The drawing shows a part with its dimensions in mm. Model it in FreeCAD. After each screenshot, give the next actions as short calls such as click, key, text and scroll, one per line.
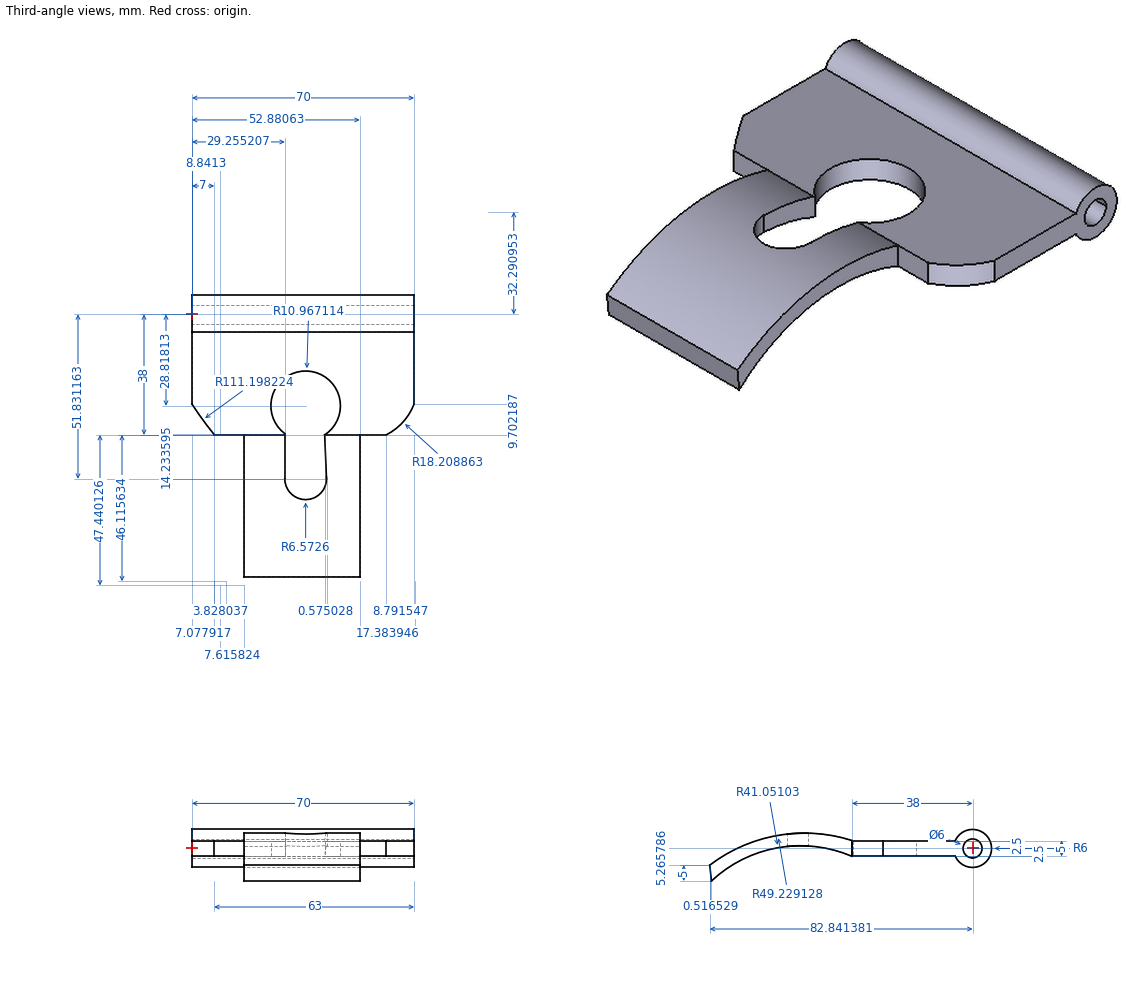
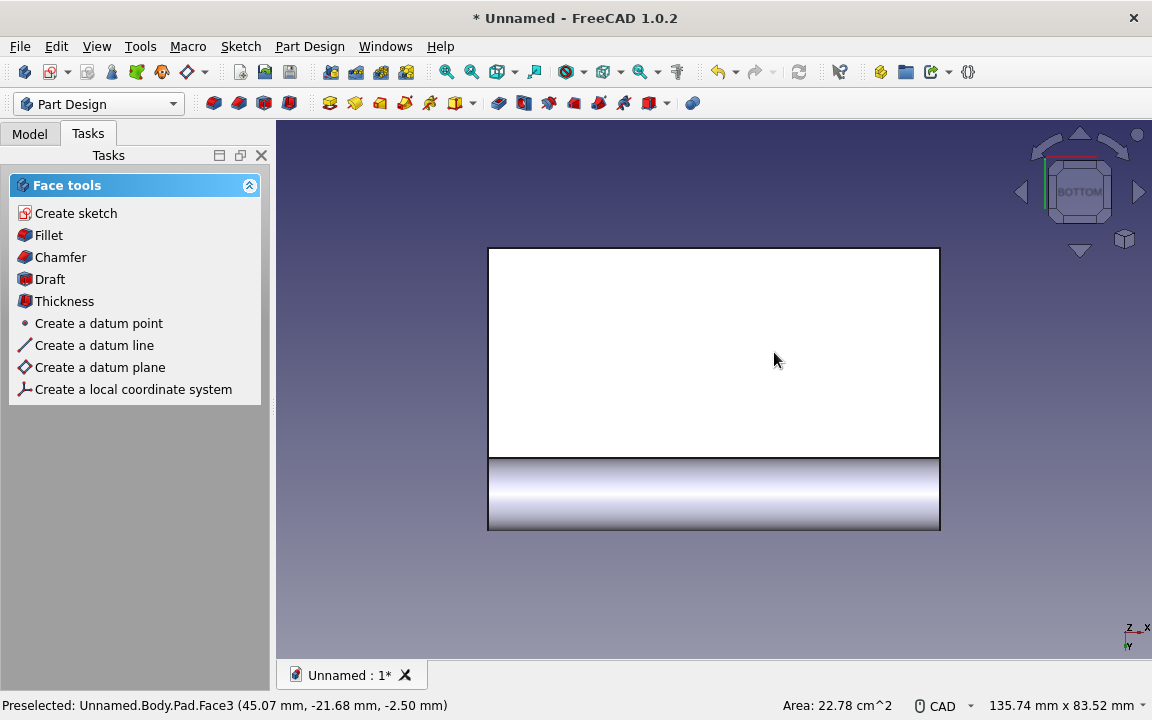
click(50, 72)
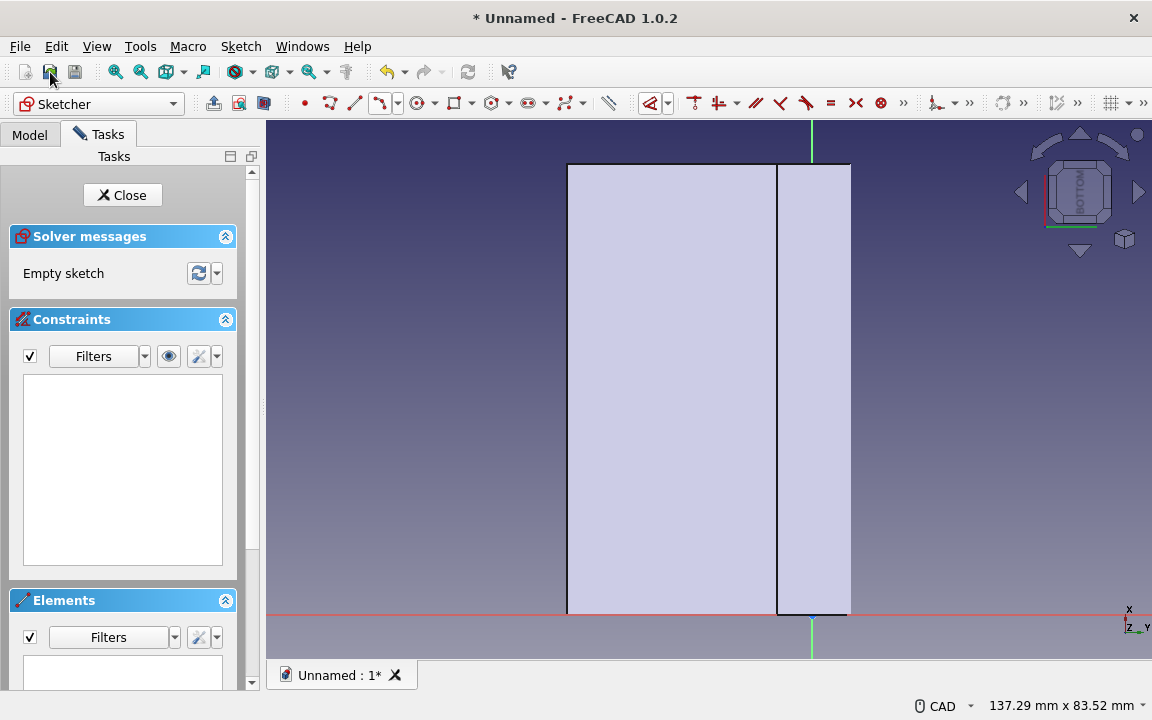
click(264, 104)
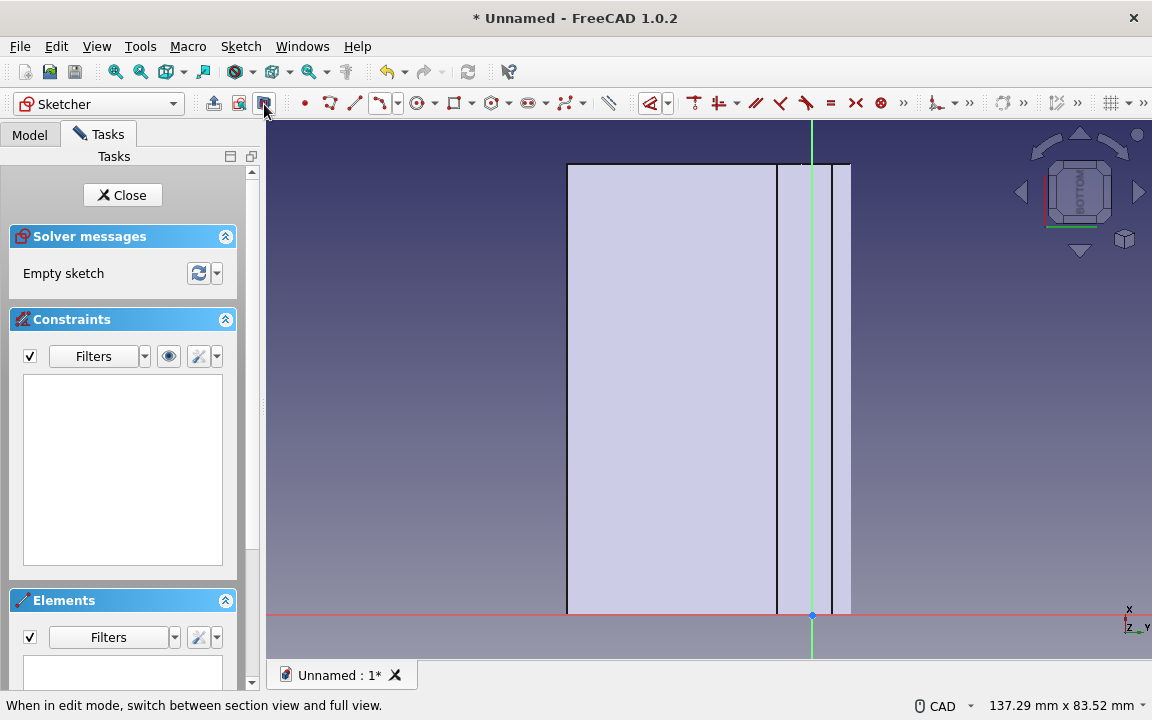
scroll(418, 389, down, 1)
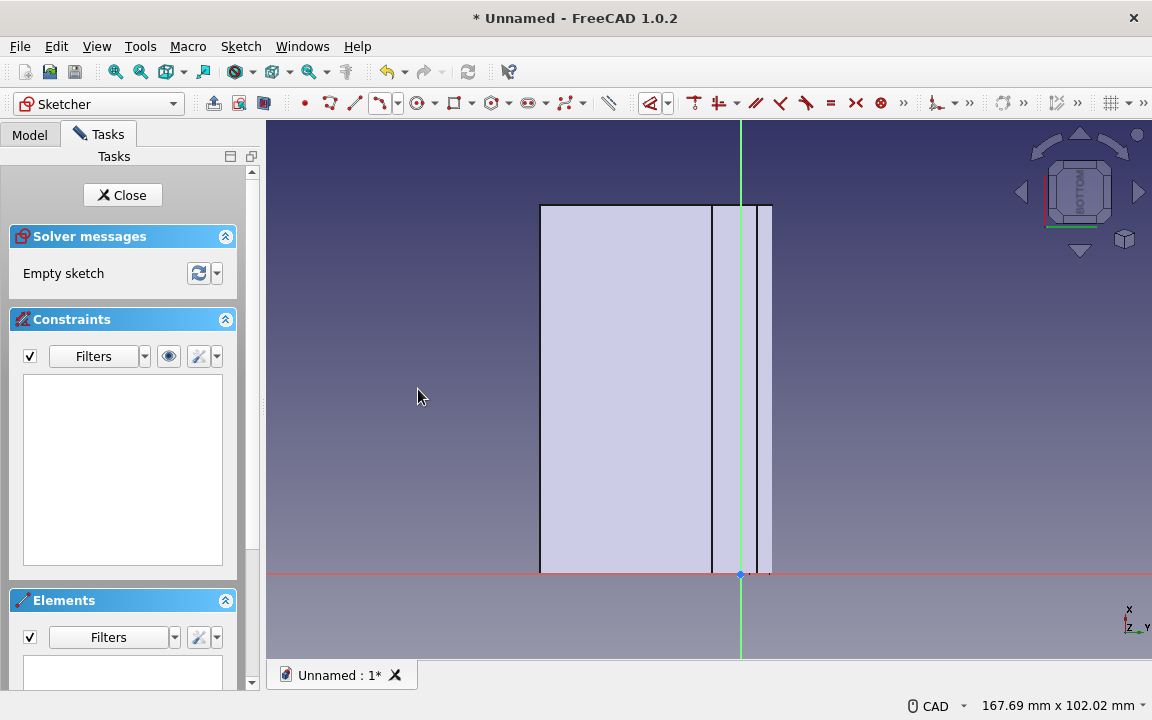
click(330, 104)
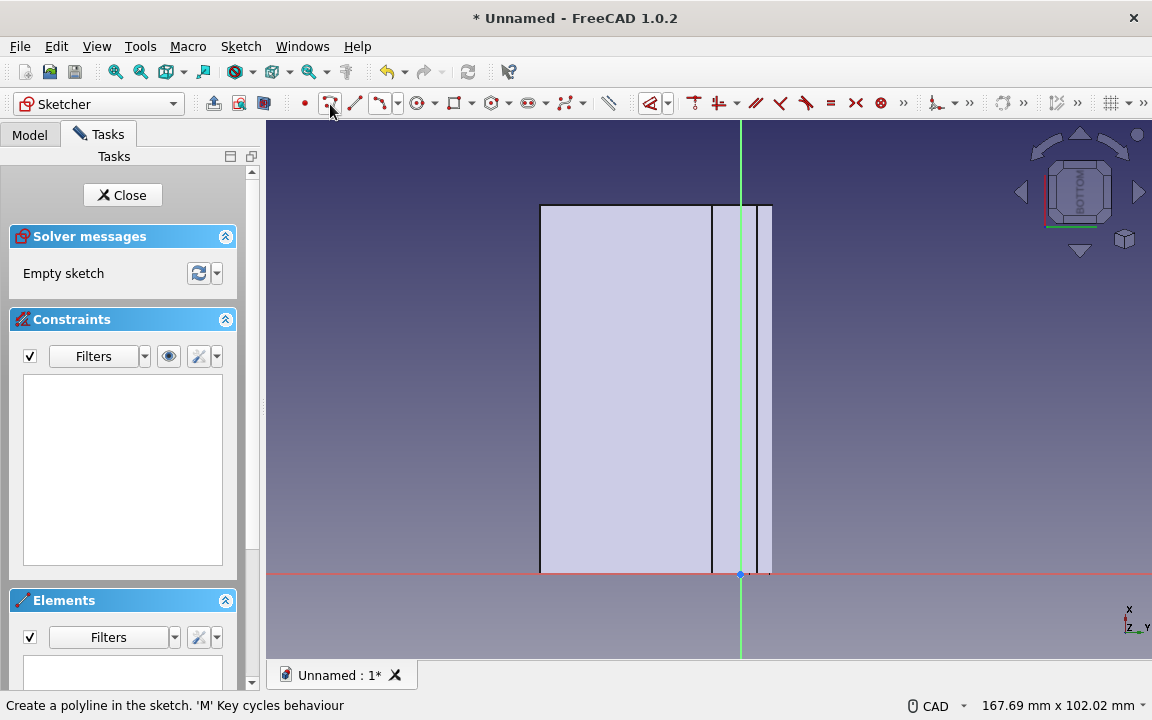
click(591, 205)
click(540, 205)
click(540, 251)
right_click(540, 251)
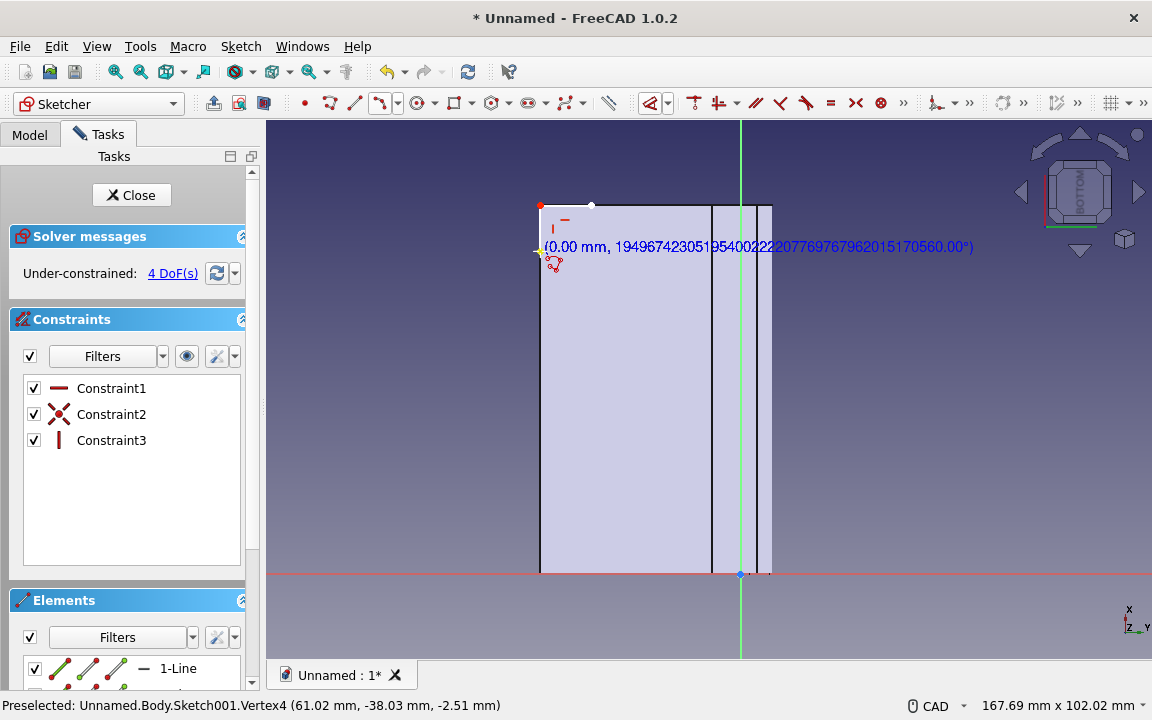
click(380, 104)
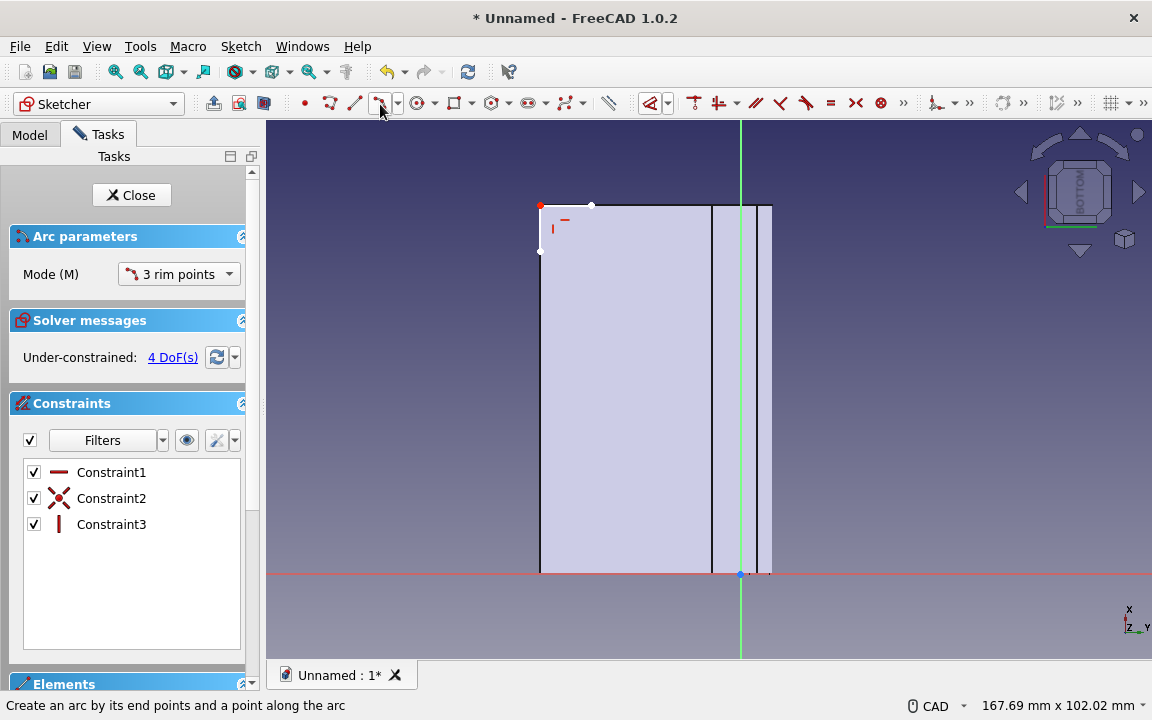
click(540, 252)
click(591, 206)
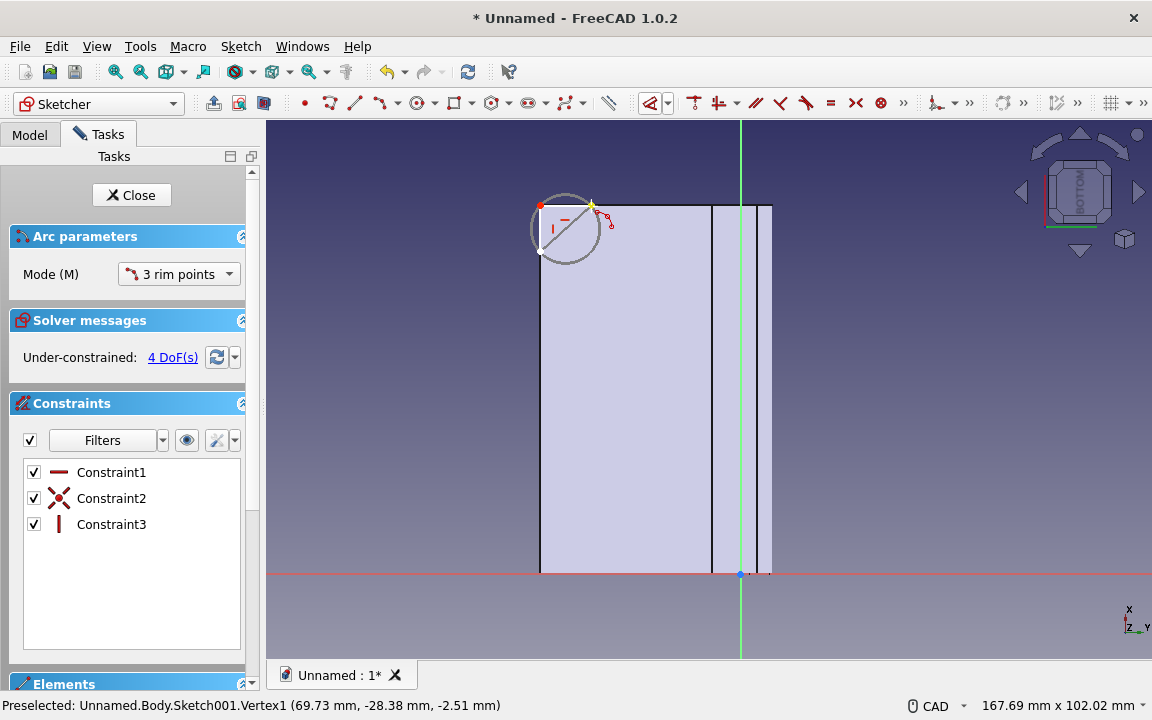
scroll(561, 223, up, 5)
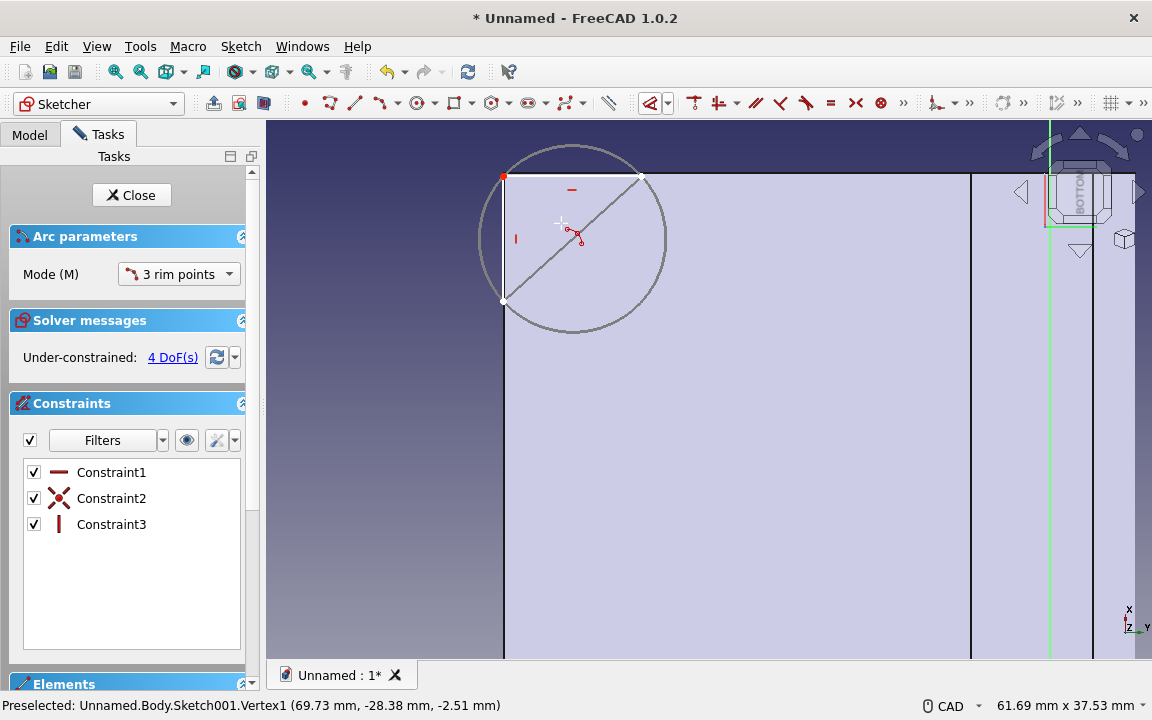
click(562, 223)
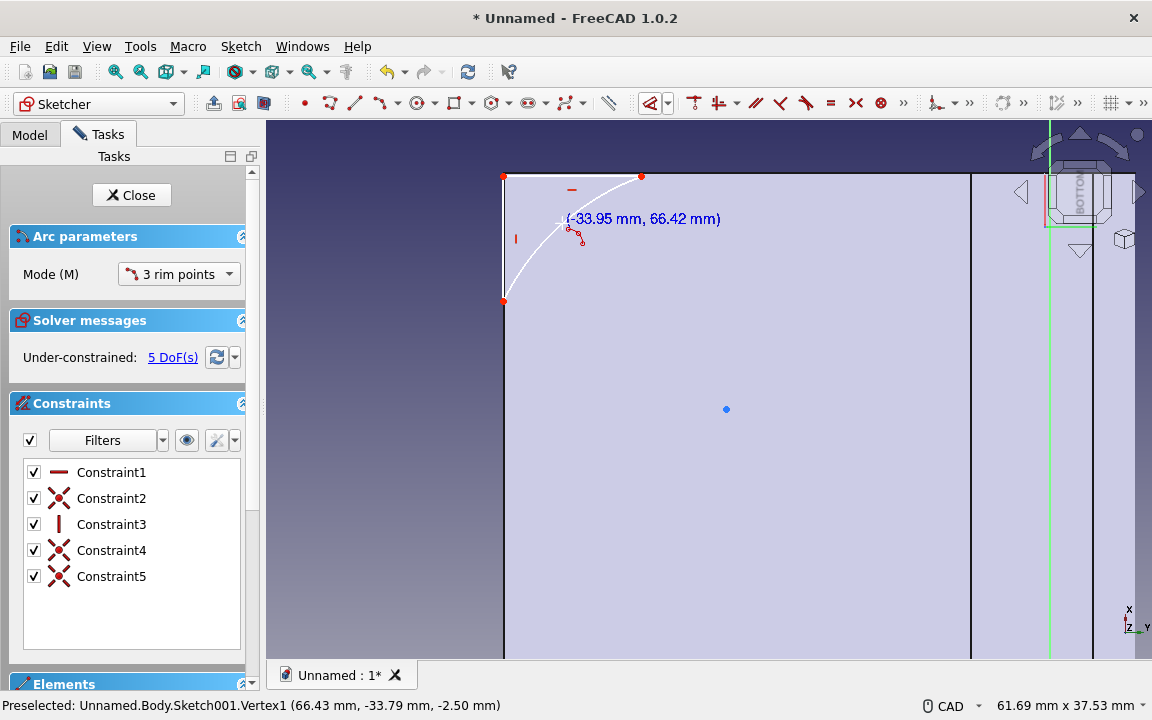
click(330, 104)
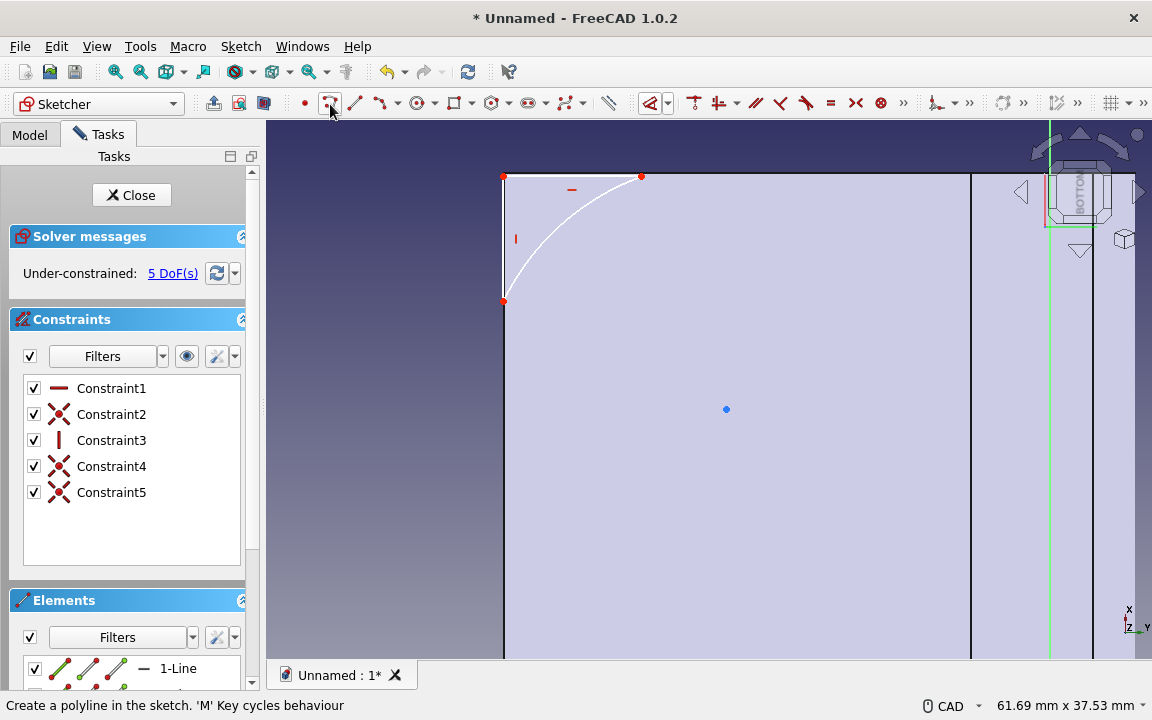
scroll(561, 223, down, 5)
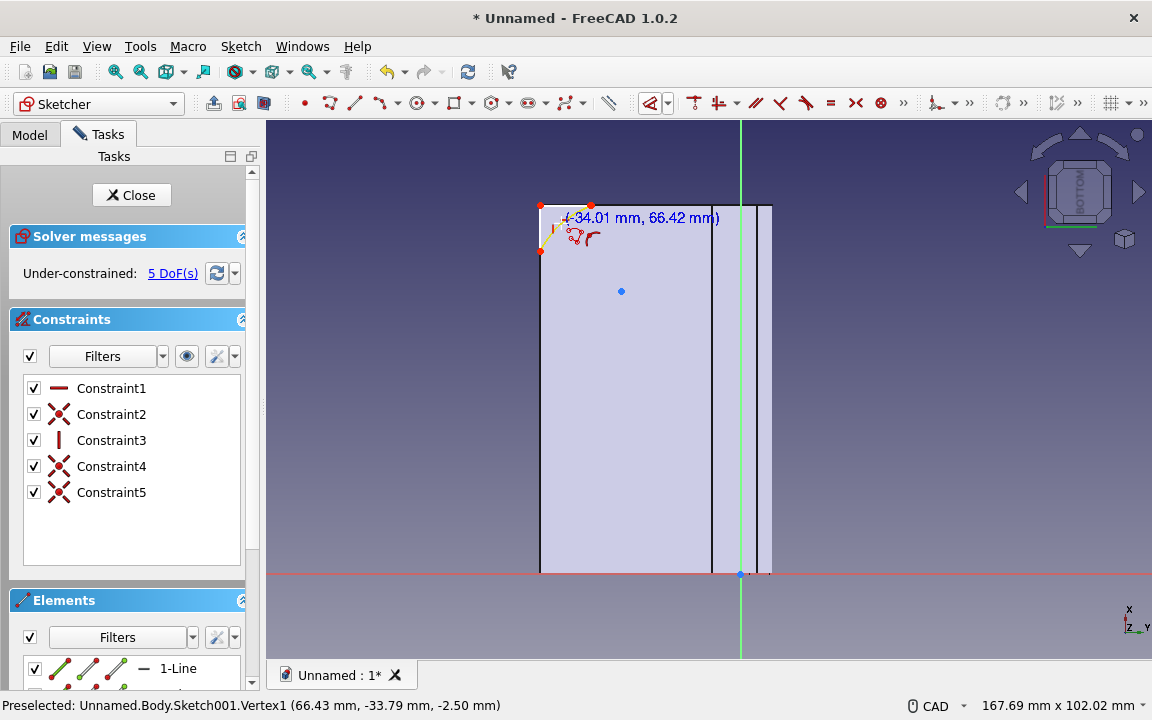
click(540, 537)
click(540, 574)
click(591, 565)
right_click(591, 565)